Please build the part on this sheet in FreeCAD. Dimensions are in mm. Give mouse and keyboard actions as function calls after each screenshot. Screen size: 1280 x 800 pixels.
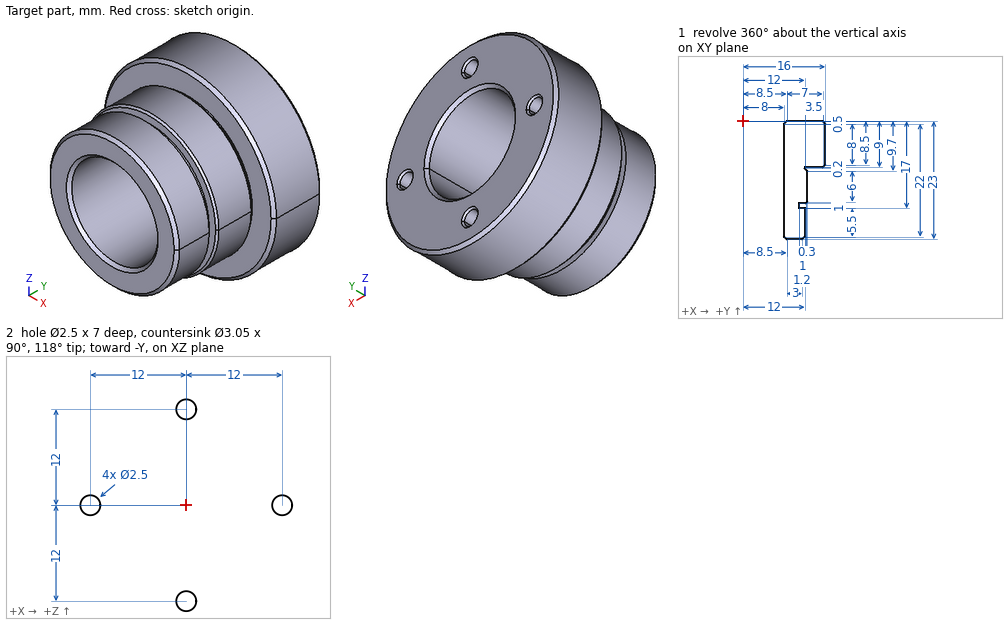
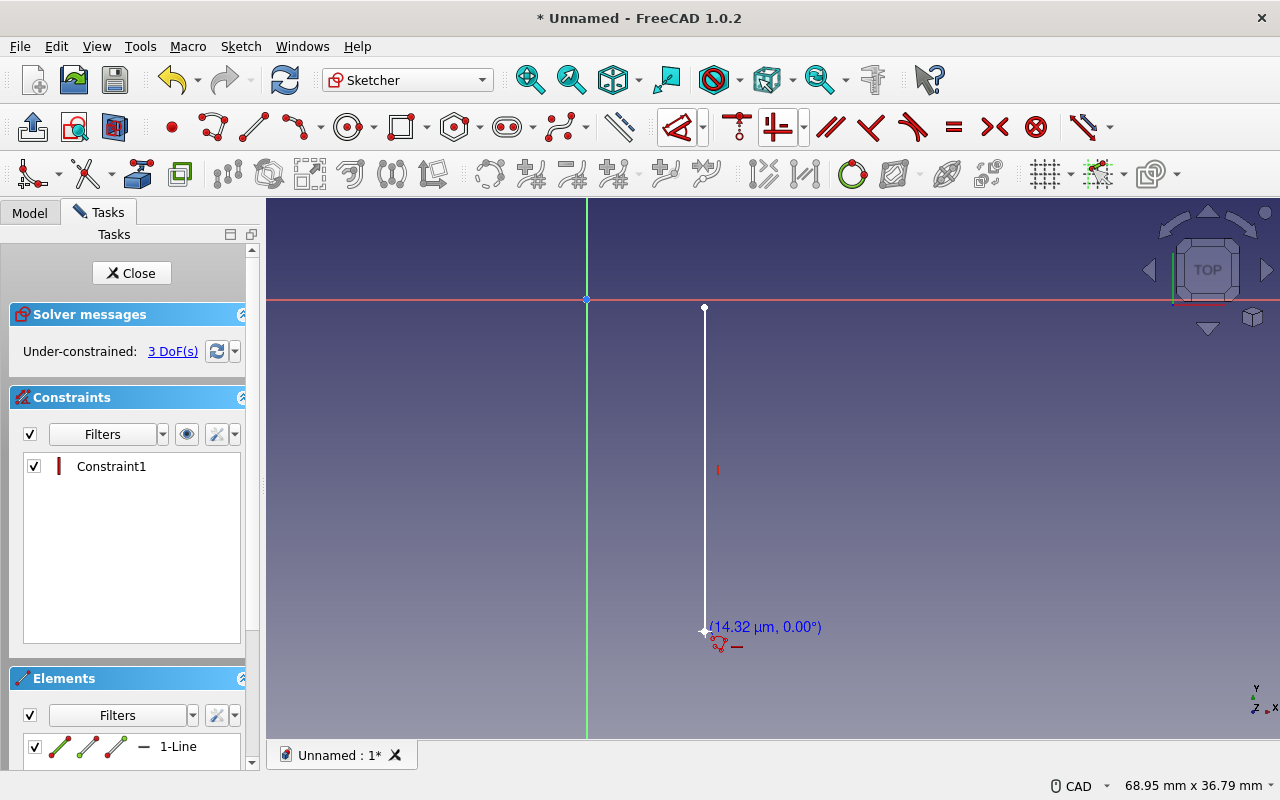
scroll(712, 638, up, 3)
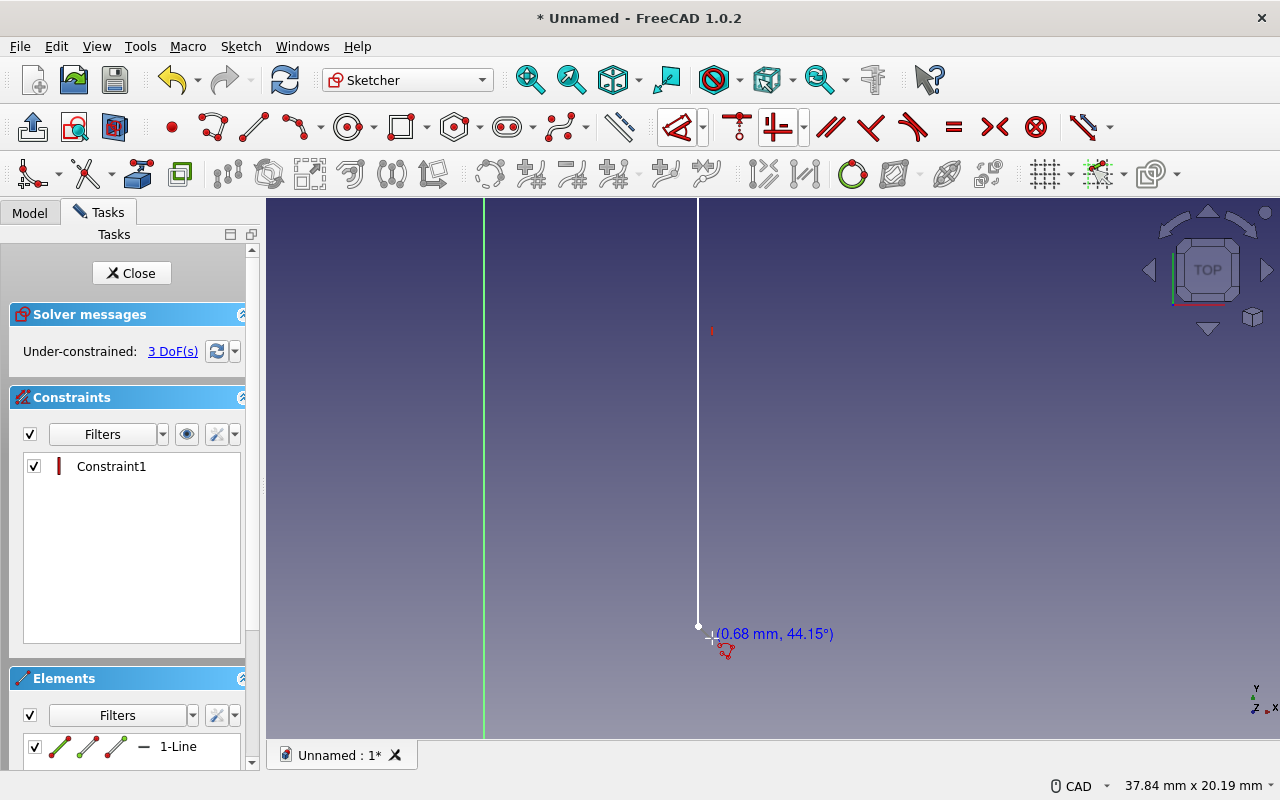
click(712, 637)
click(792, 637)
click(805, 624)
click(805, 476)
click(779, 476)
click(779, 450)
click(811, 450)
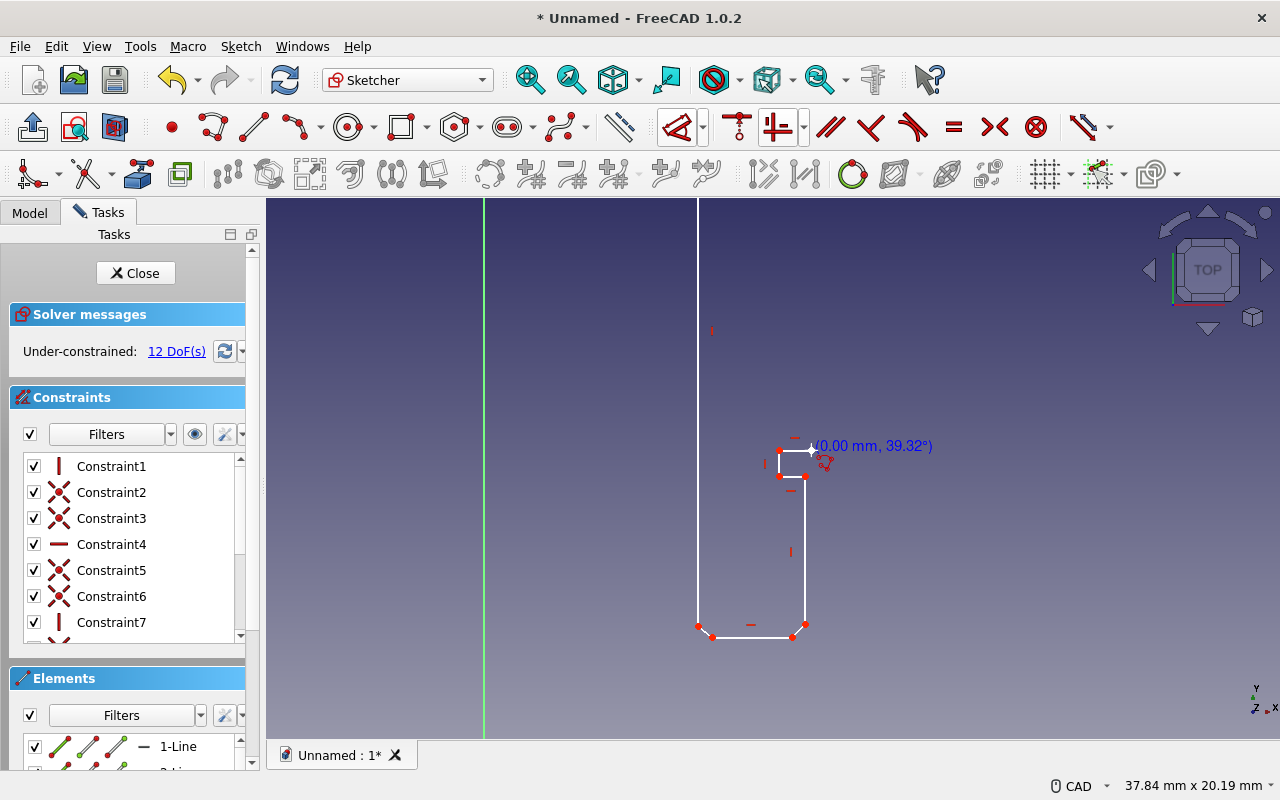
scroll(819, 442, up, 2)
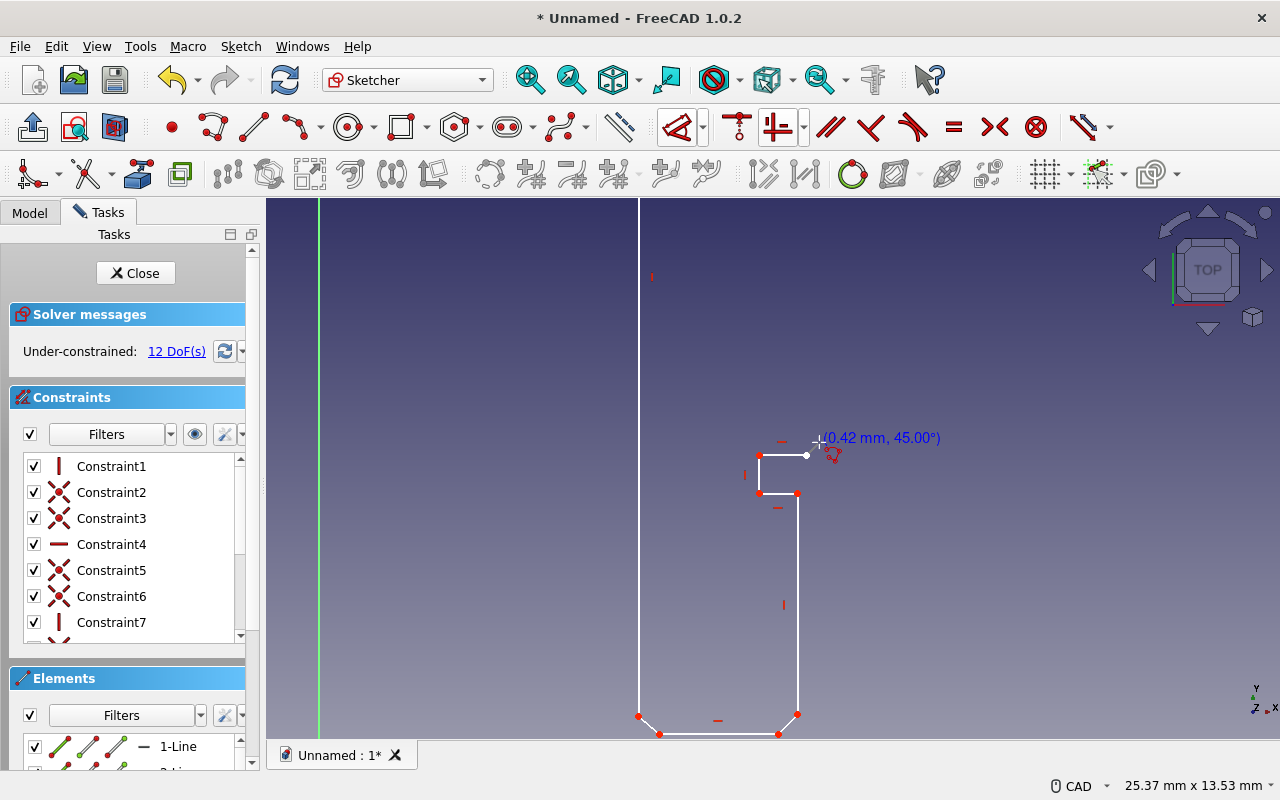
click(818, 441)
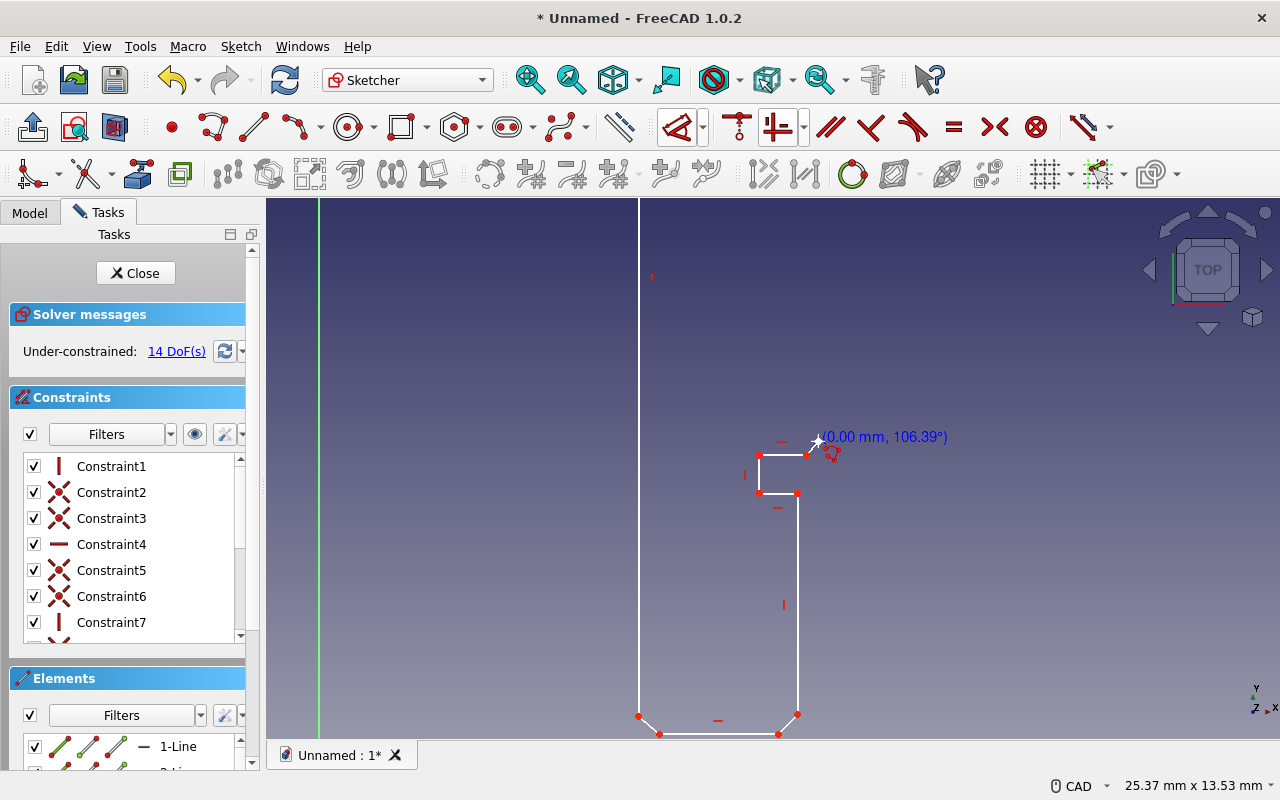
scroll(743, 582, down, 5)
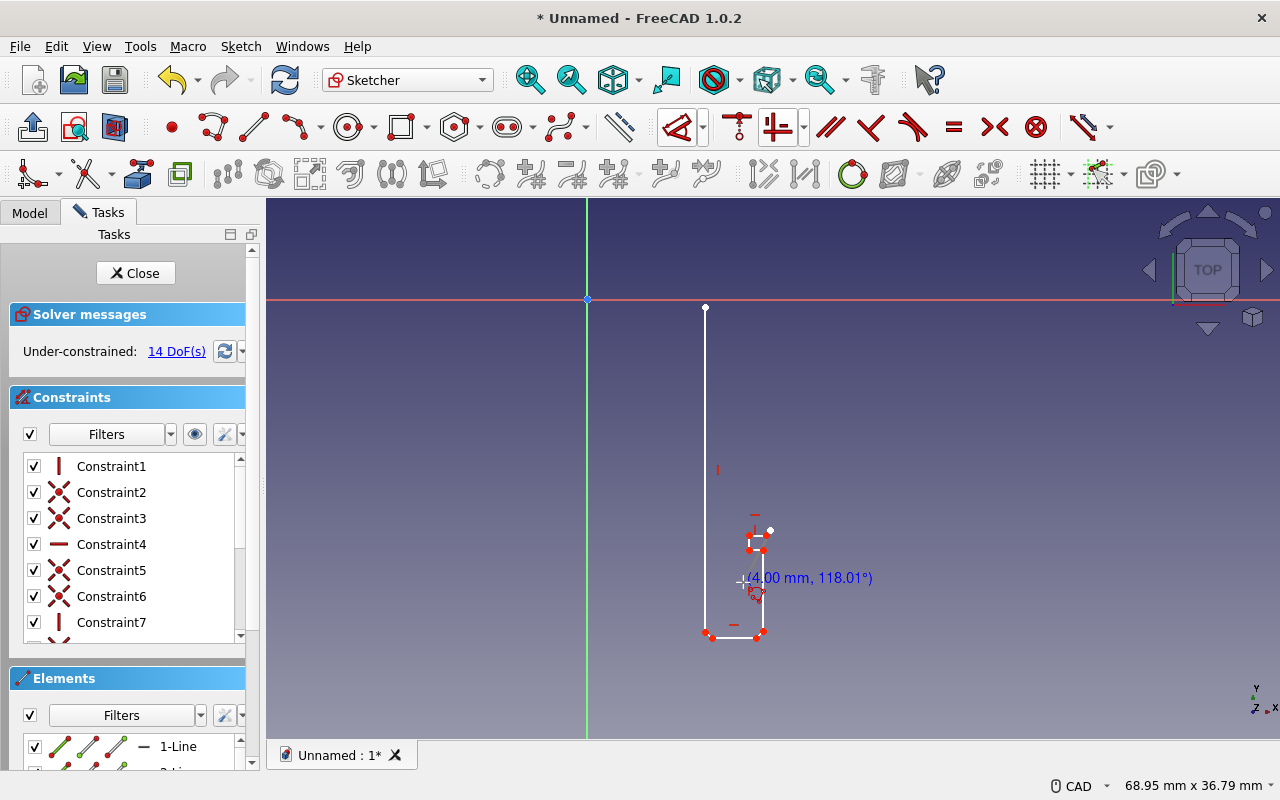
click(771, 442)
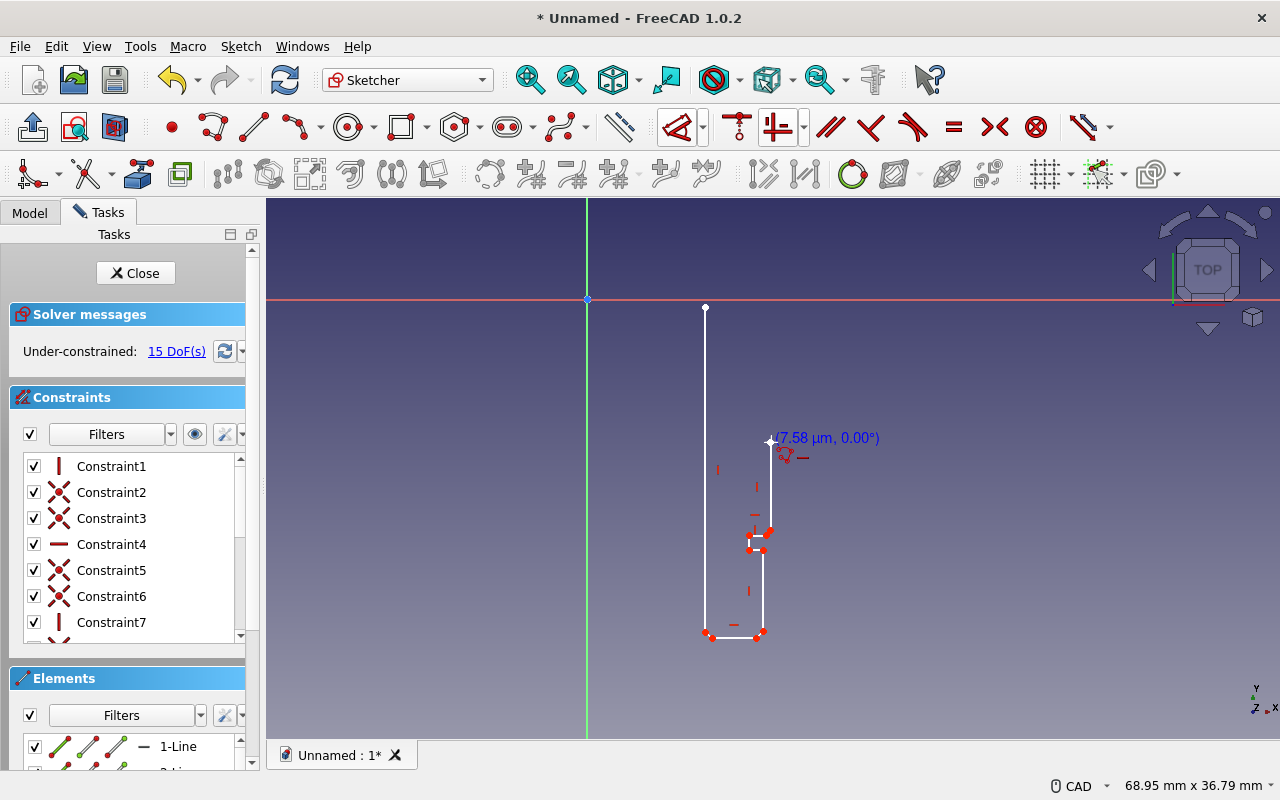
scroll(764, 435, up, 3)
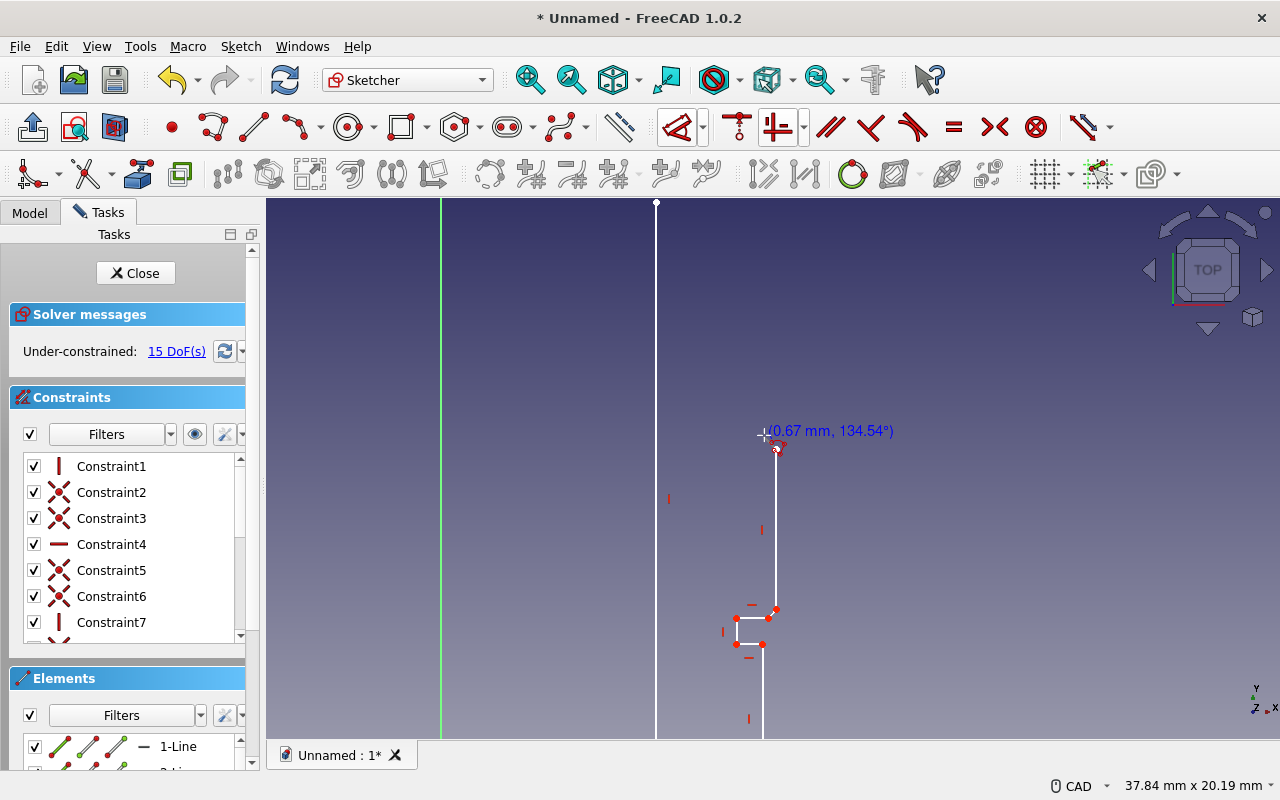
click(763, 435)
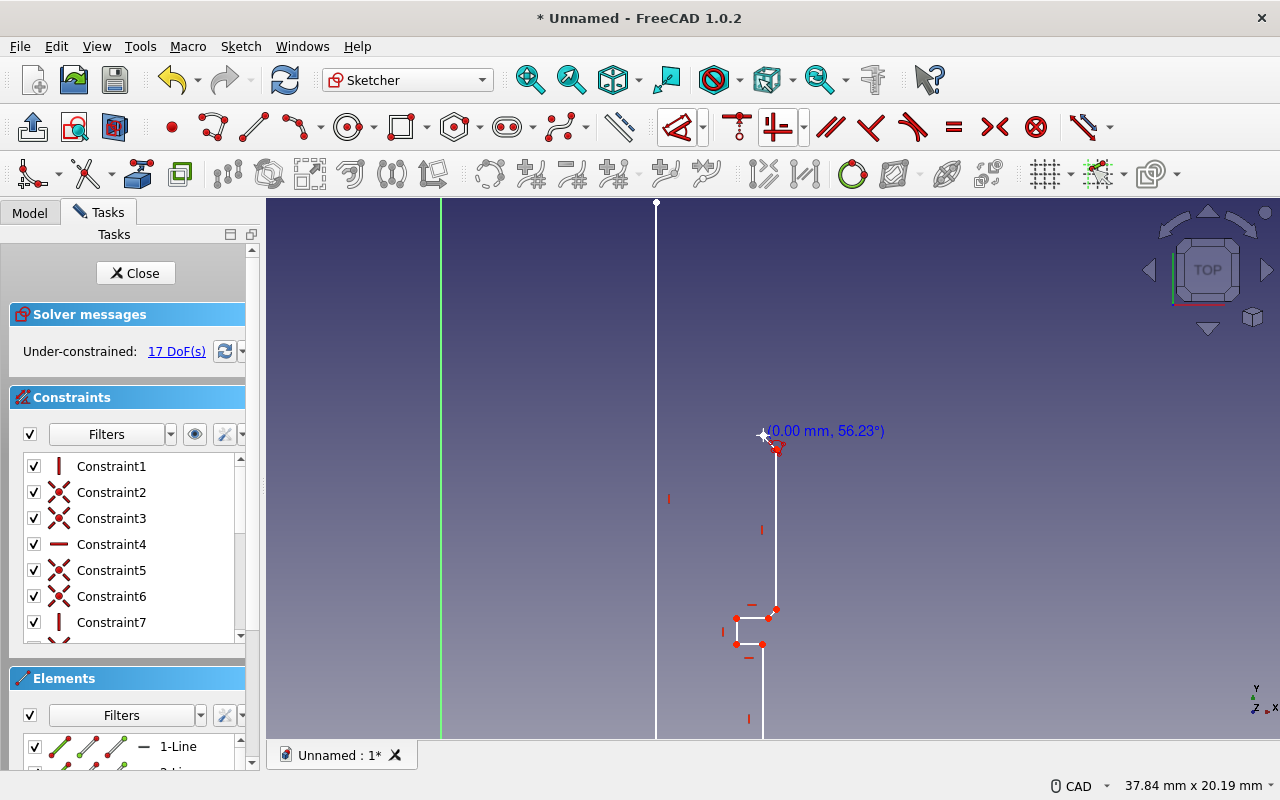
scroll(763, 429, up, 6)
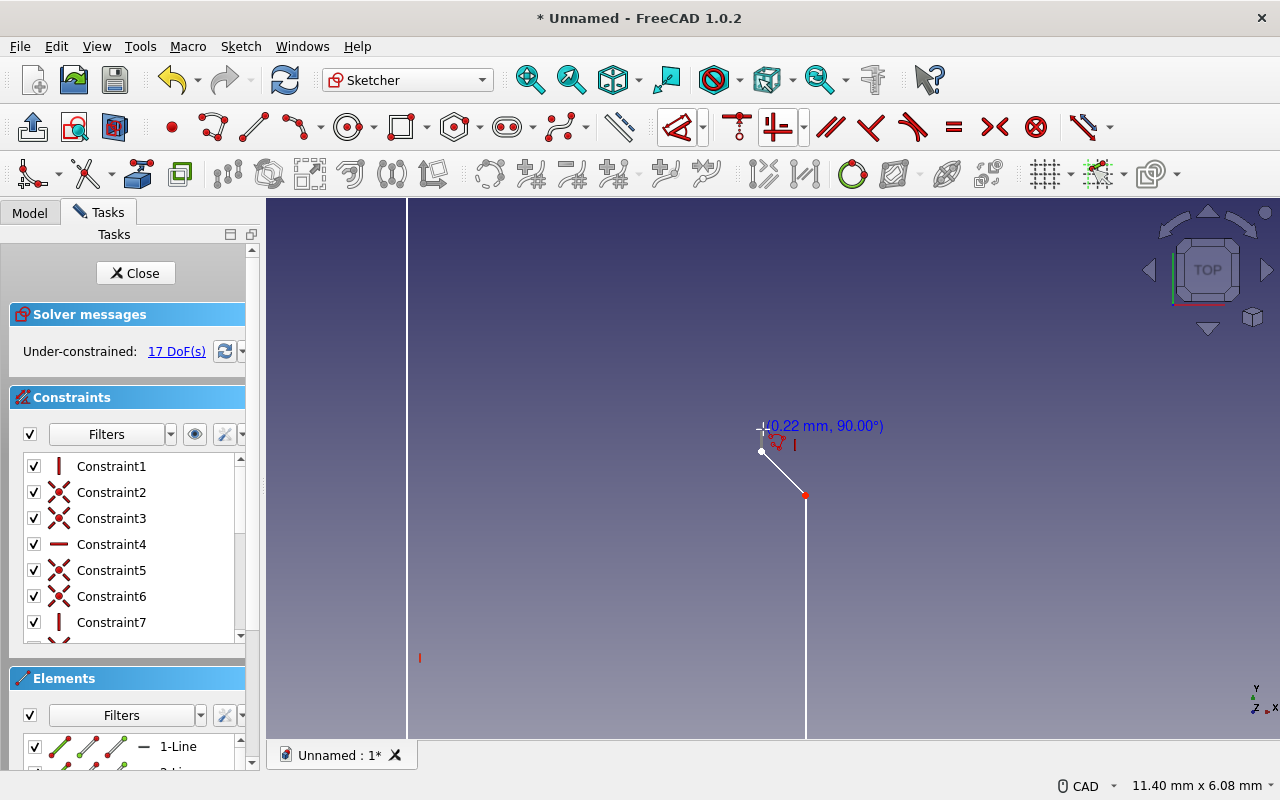
click(762, 429)